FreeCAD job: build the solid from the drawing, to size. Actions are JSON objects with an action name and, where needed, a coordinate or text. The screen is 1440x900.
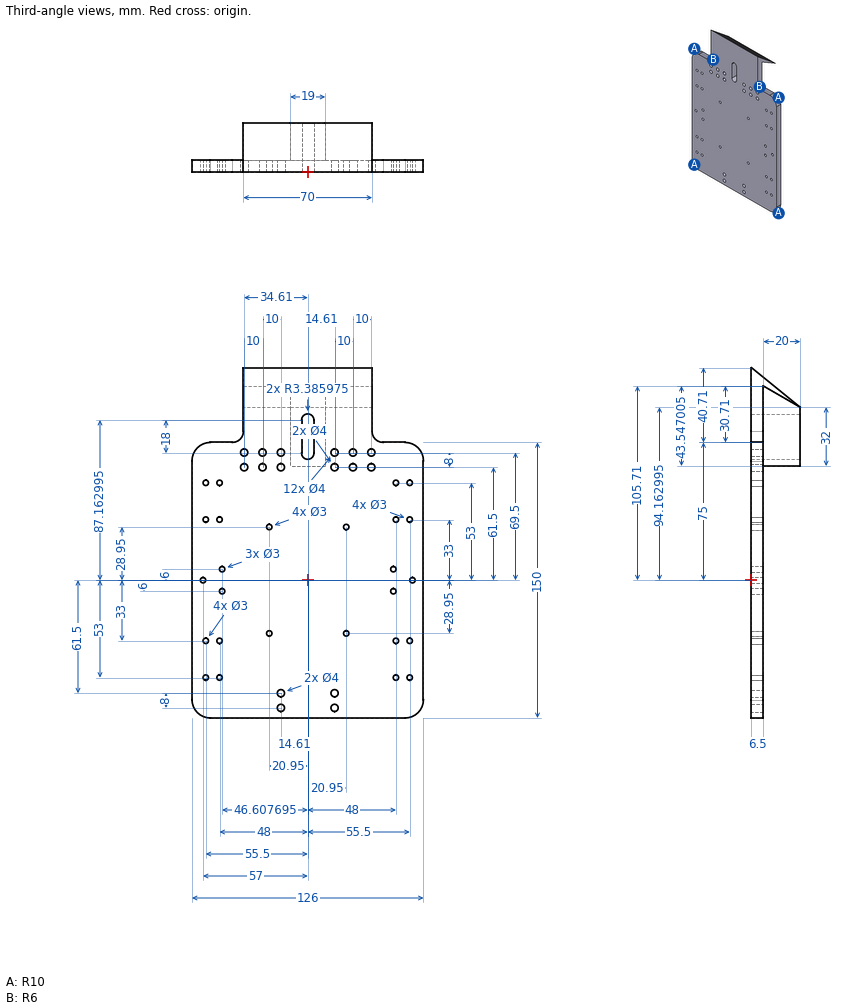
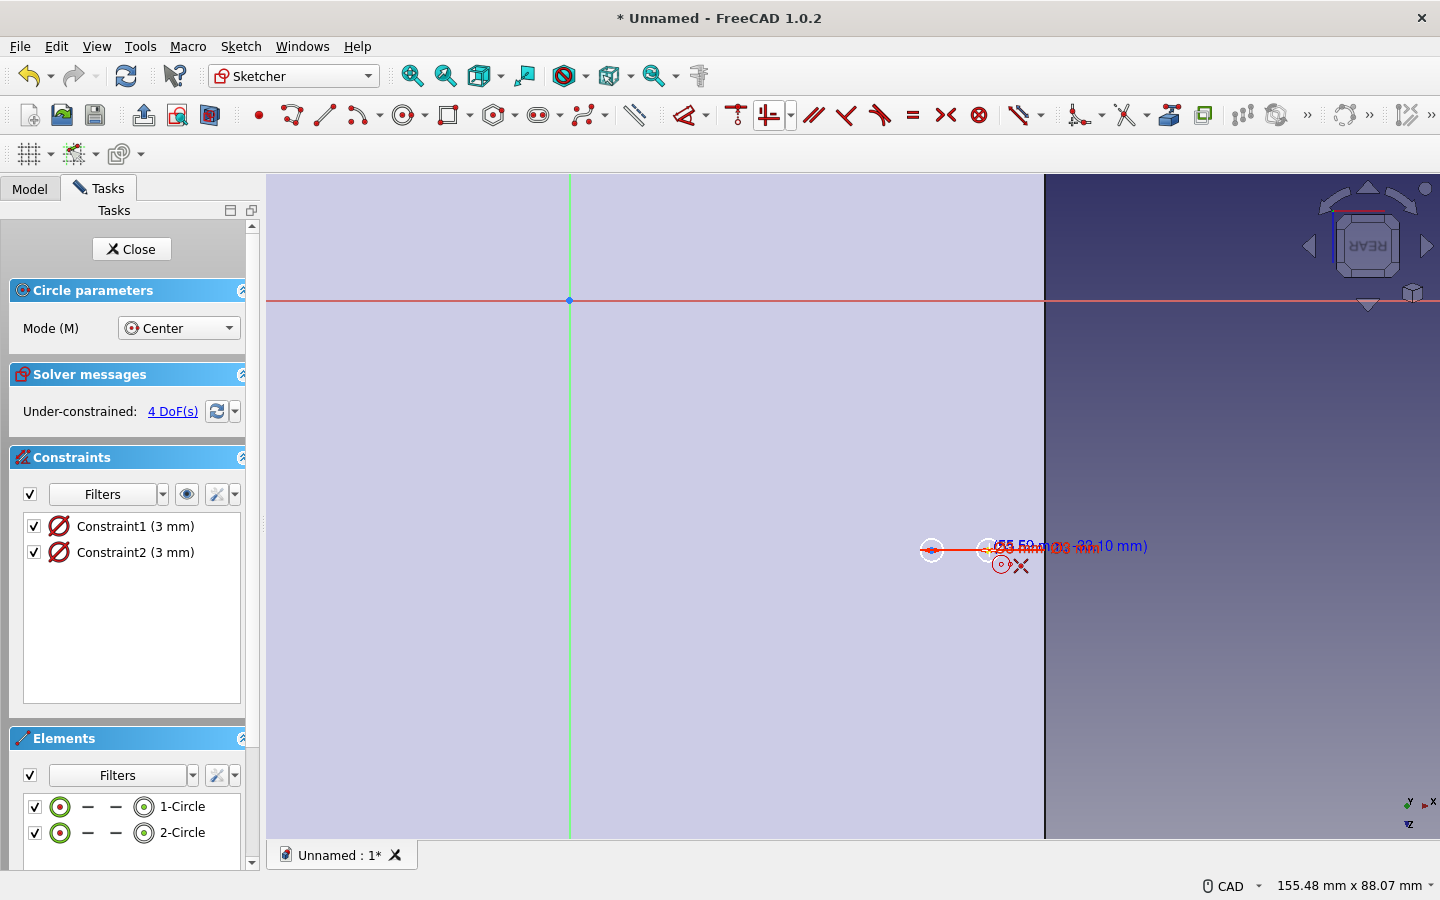
{"action": "scroll", "coordinate": [932, 701], "scroll_direction": "up", "scroll_amount": 4}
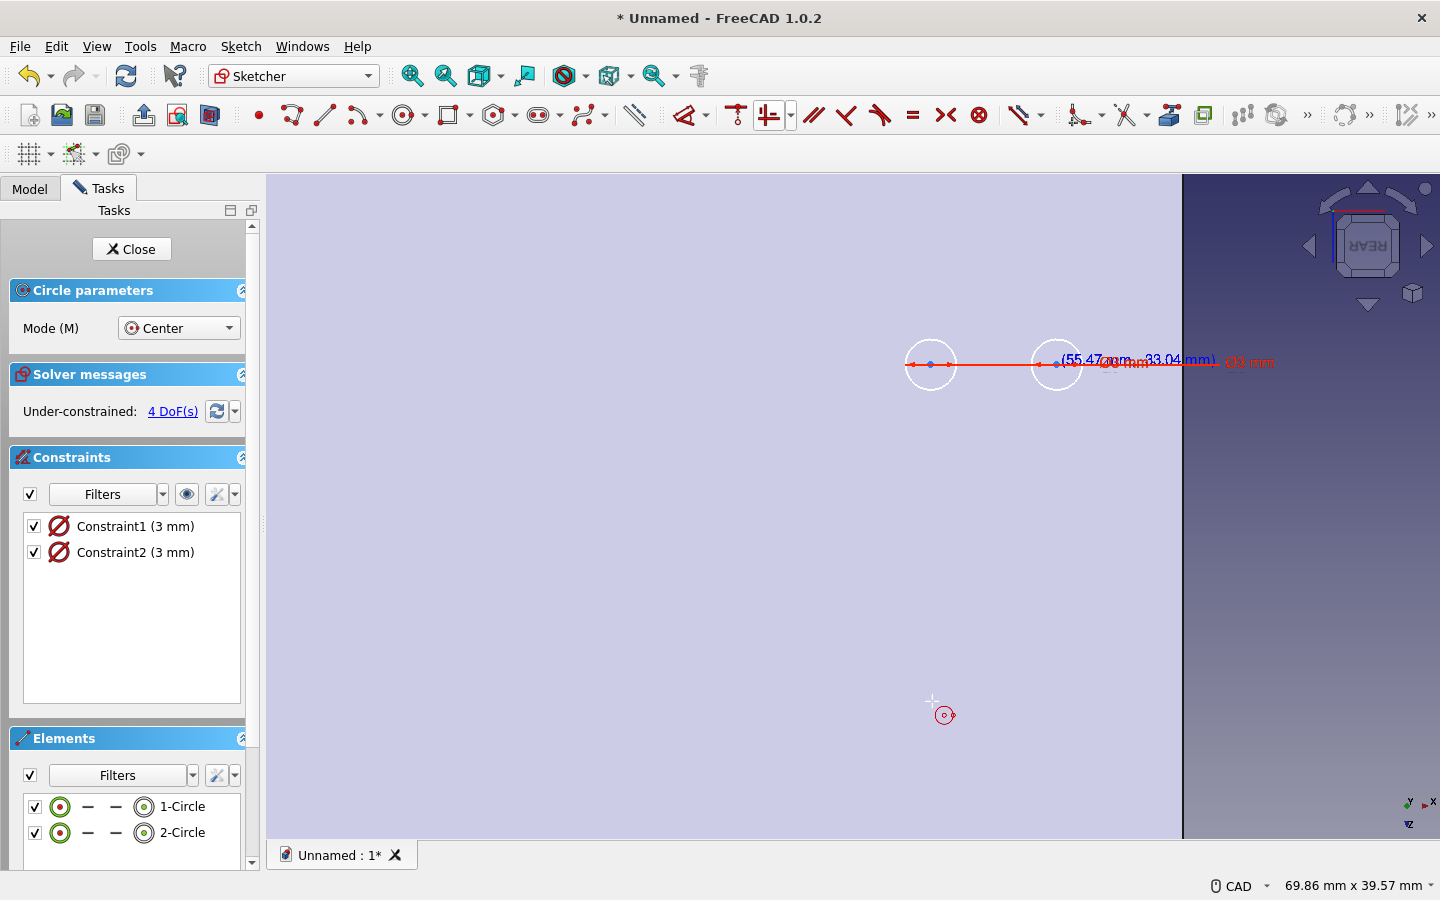
{"action": "left_click", "coordinate": [931, 700]}
{"action": "mouse_move", "coordinate": [949, 682]}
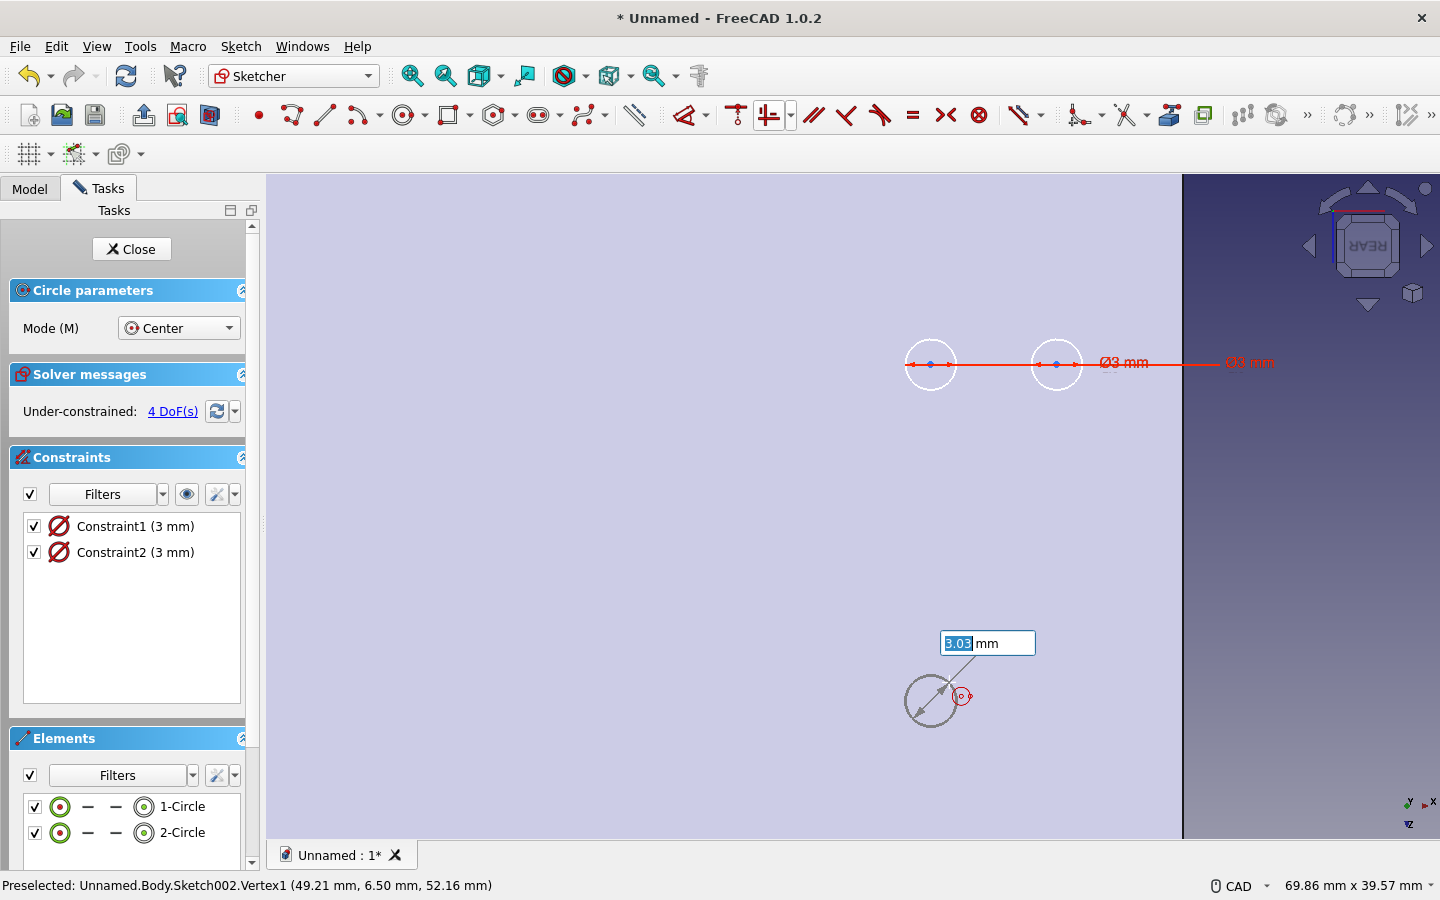
{"action": "type", "text": "3"}
{"action": "key", "text": "Return"}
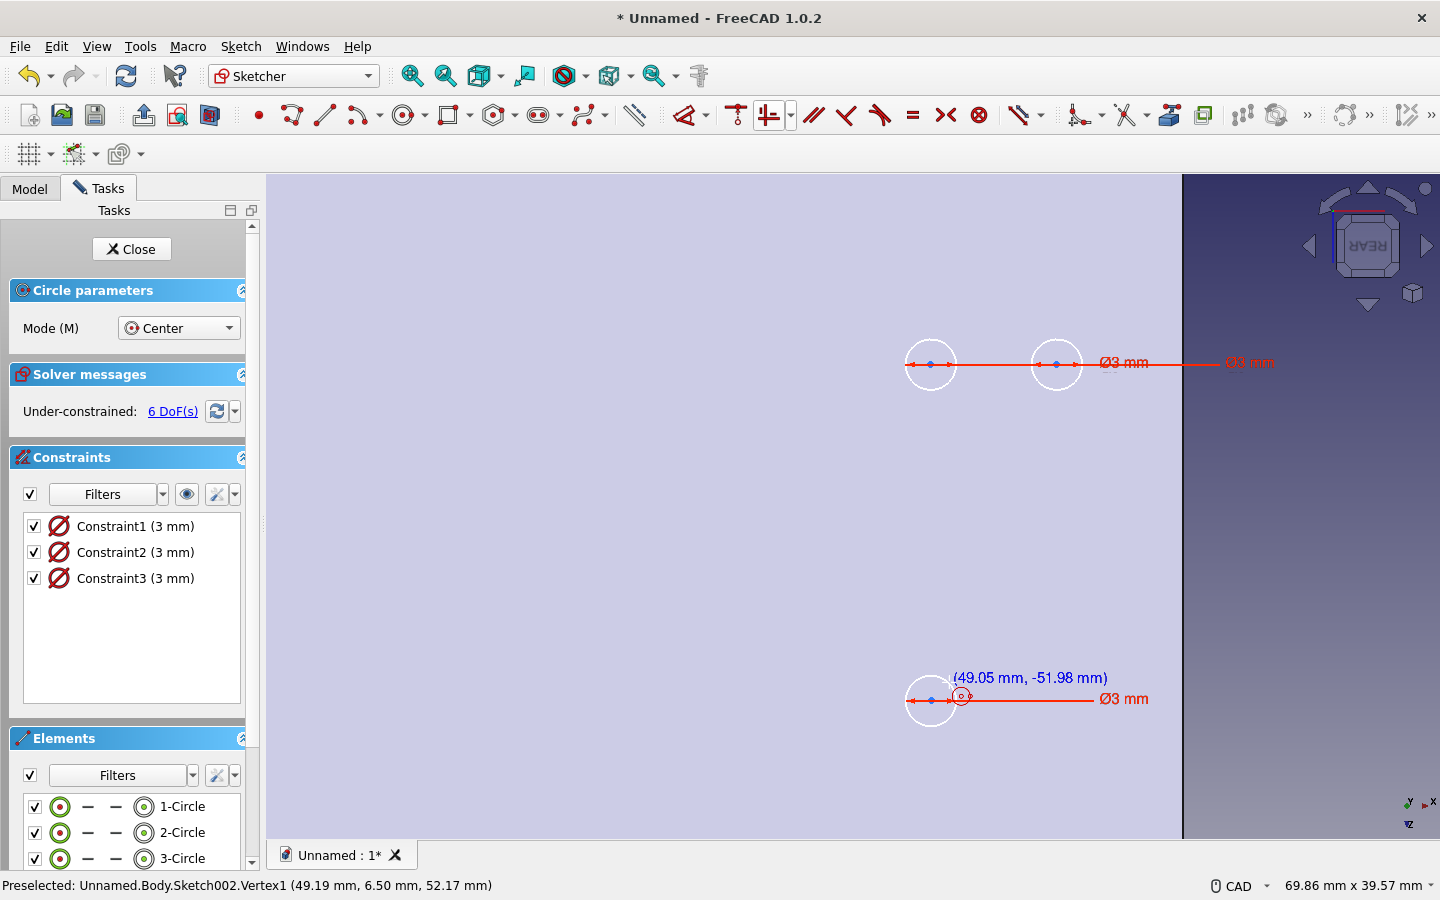
{"action": "left_click", "coordinate": [1057, 700]}
{"action": "mouse_move", "coordinate": [1075, 682]}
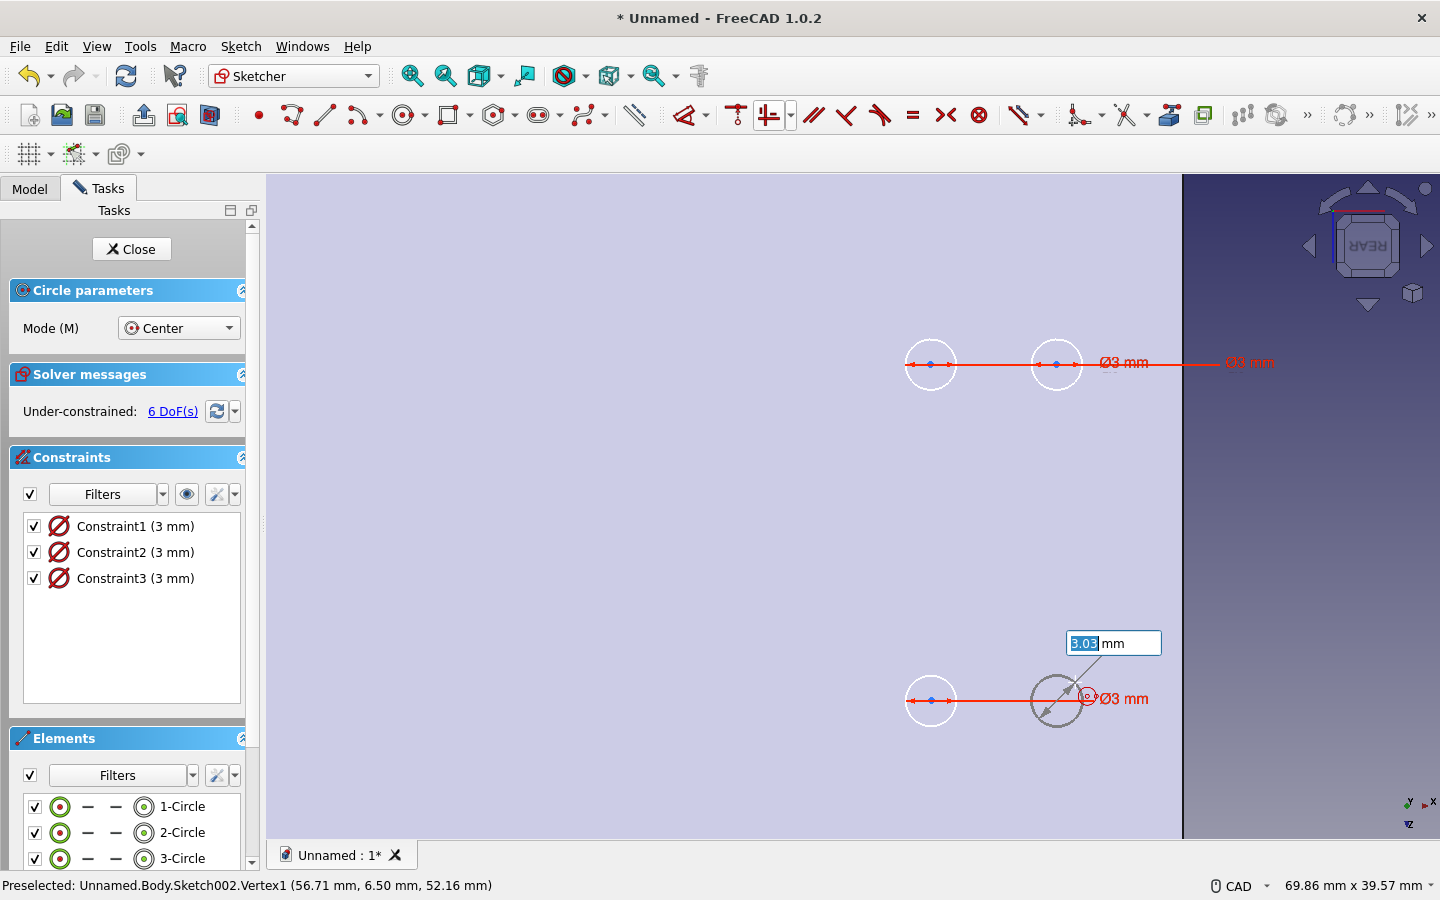
{"action": "type", "text": "3"}
{"action": "key", "text": "Return"}
{"action": "key", "text": "Escape"}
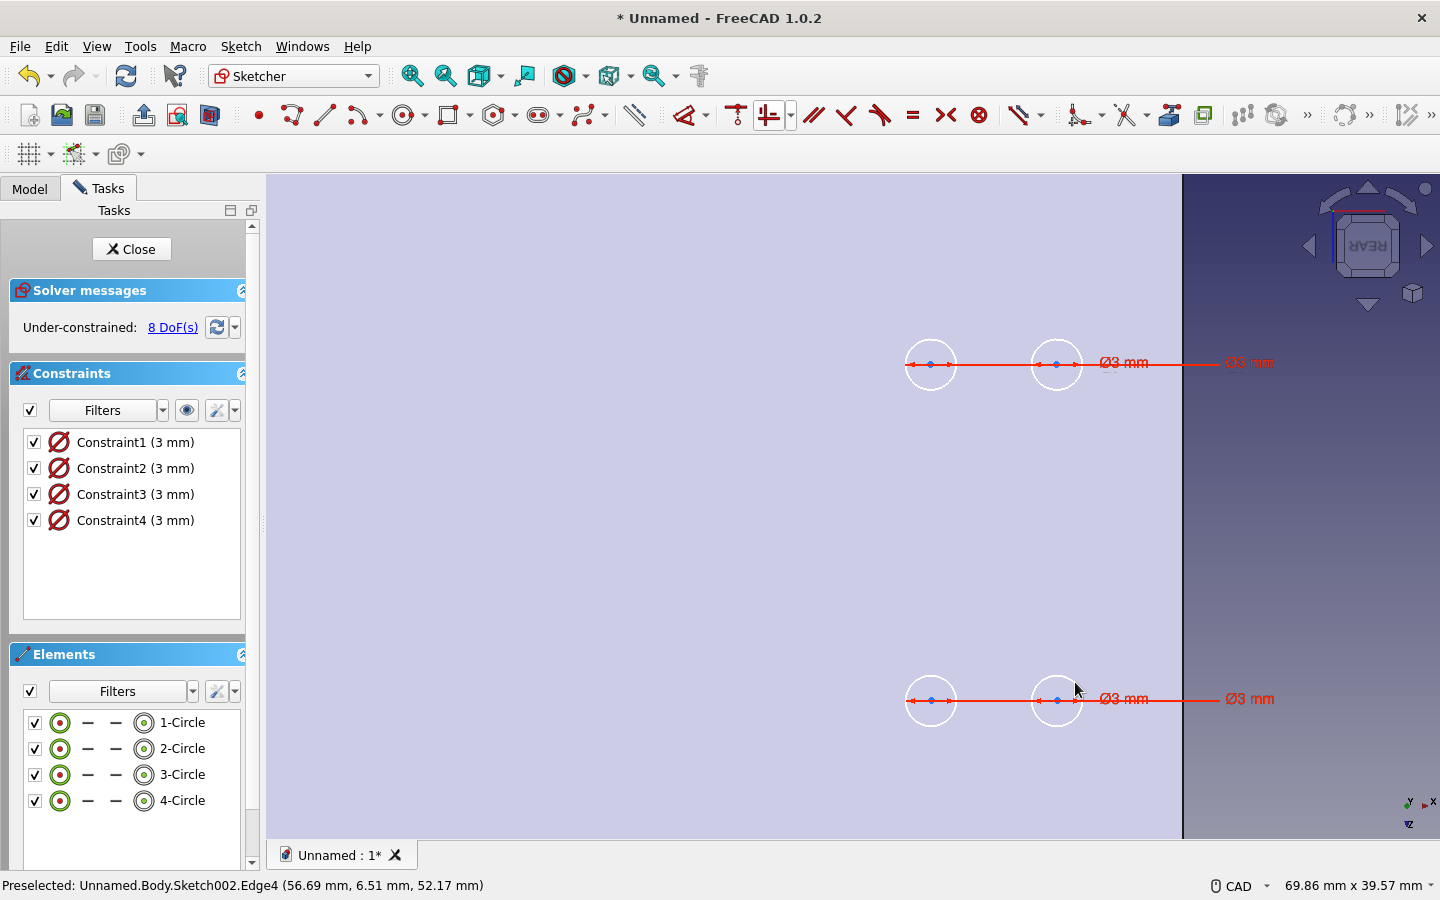
{"action": "left_click", "coordinate": [1057, 365]}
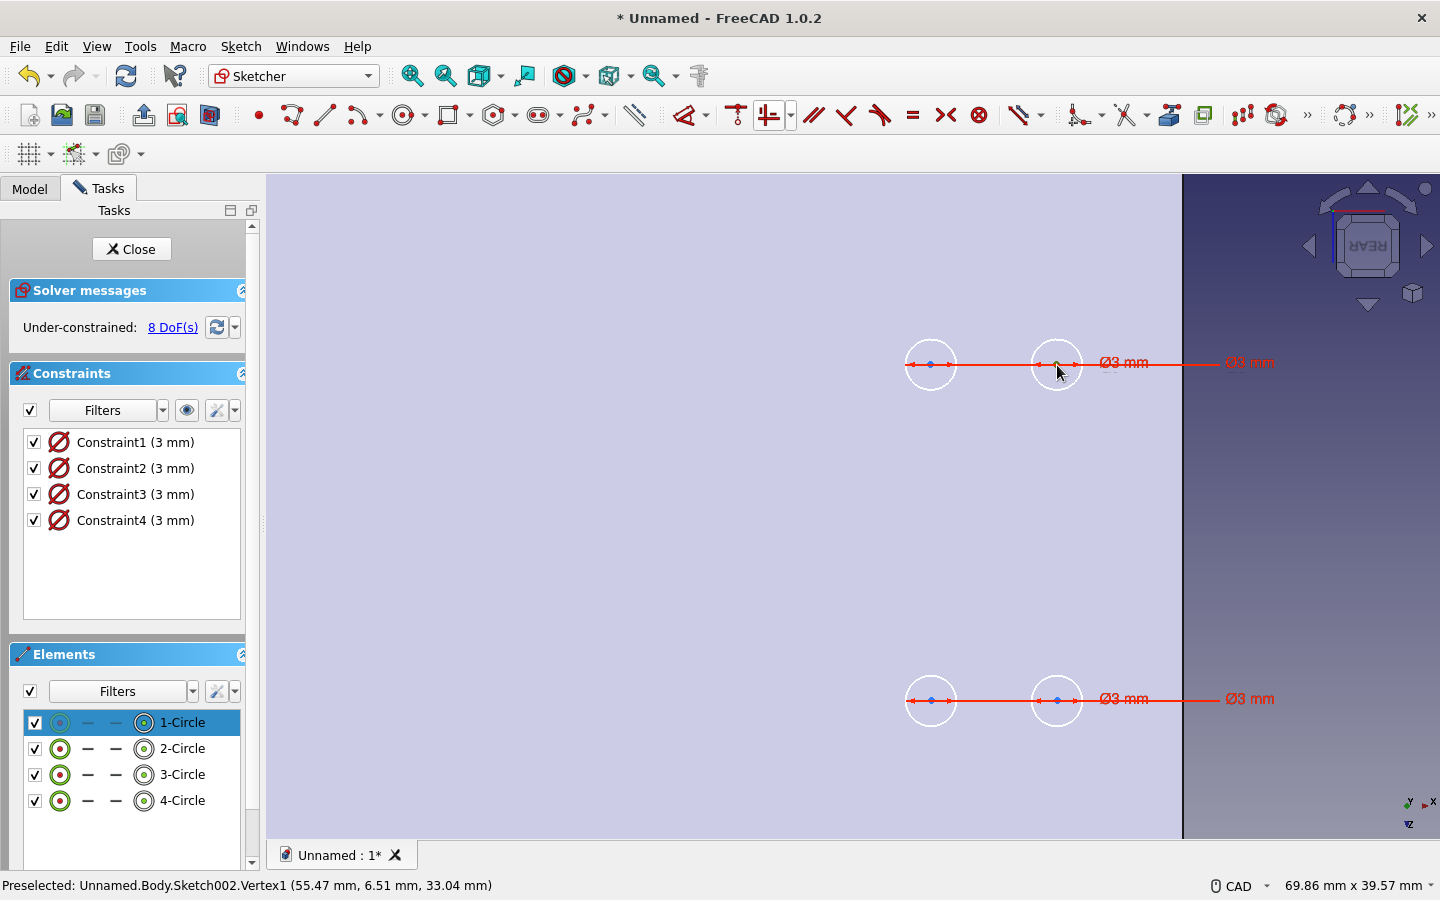
{"action": "left_click", "coordinate": [931, 365]}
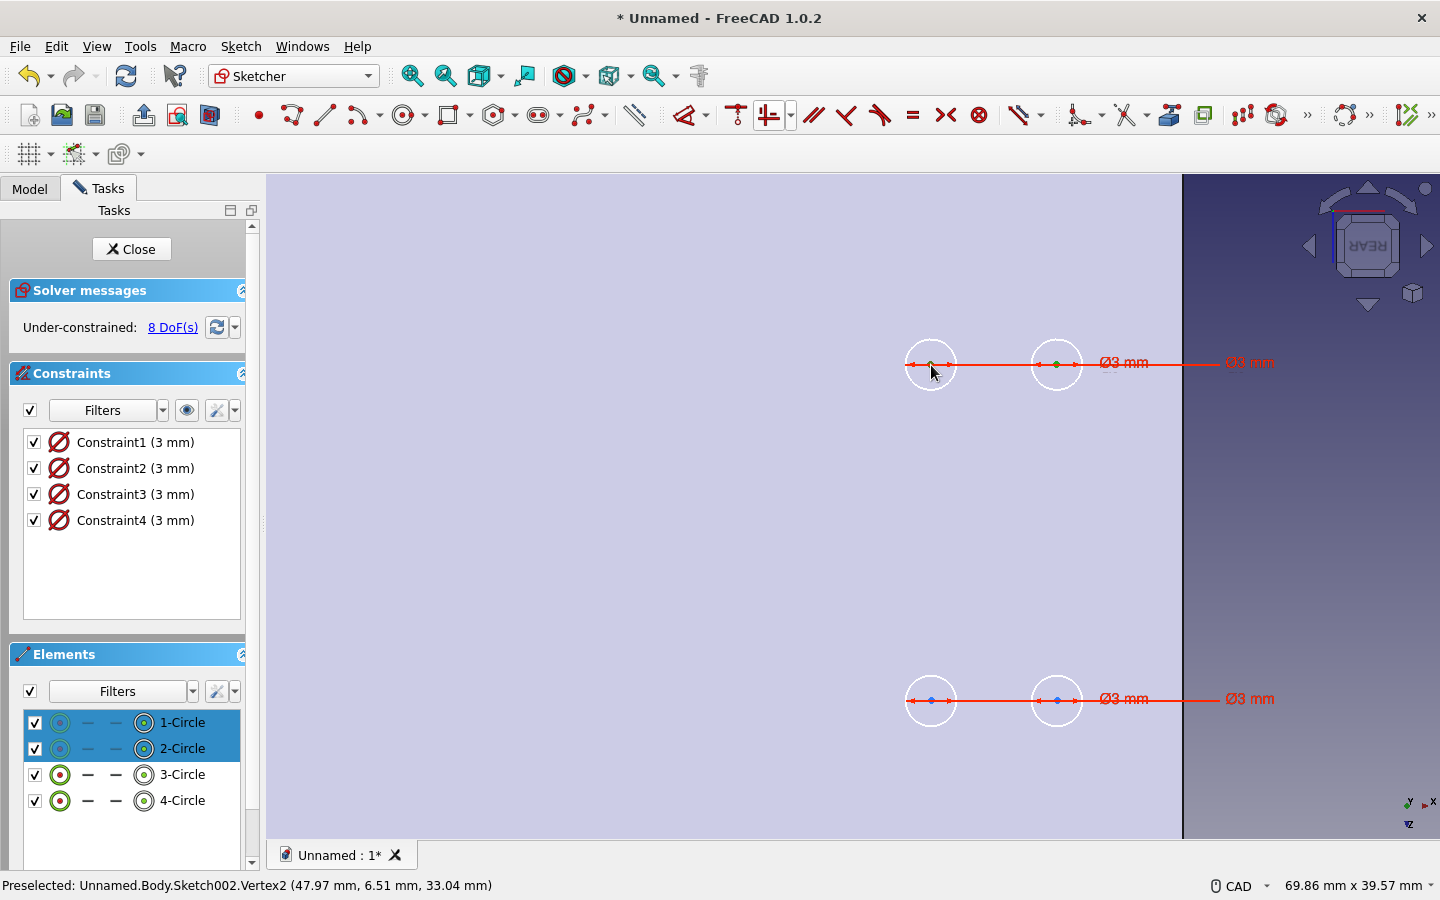
{"action": "left_click", "coordinate": [790, 116]}